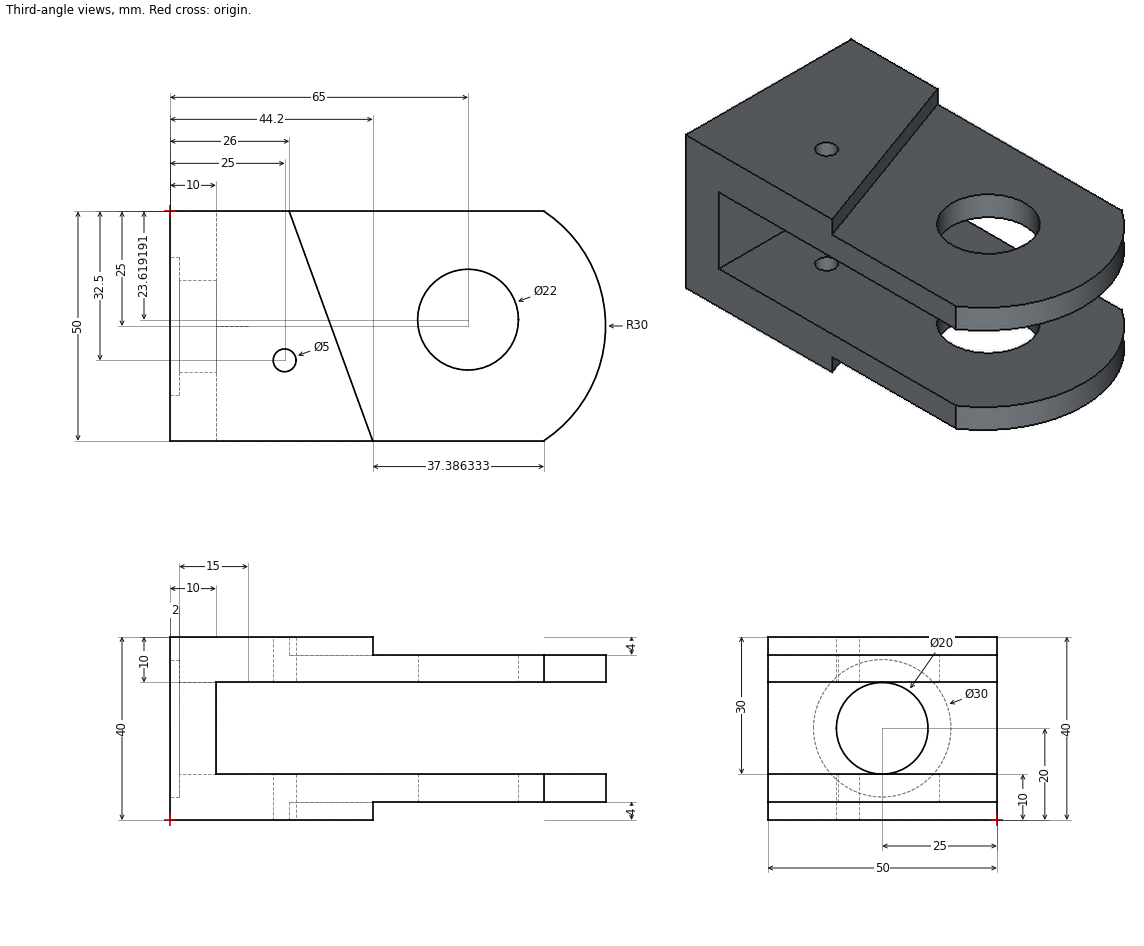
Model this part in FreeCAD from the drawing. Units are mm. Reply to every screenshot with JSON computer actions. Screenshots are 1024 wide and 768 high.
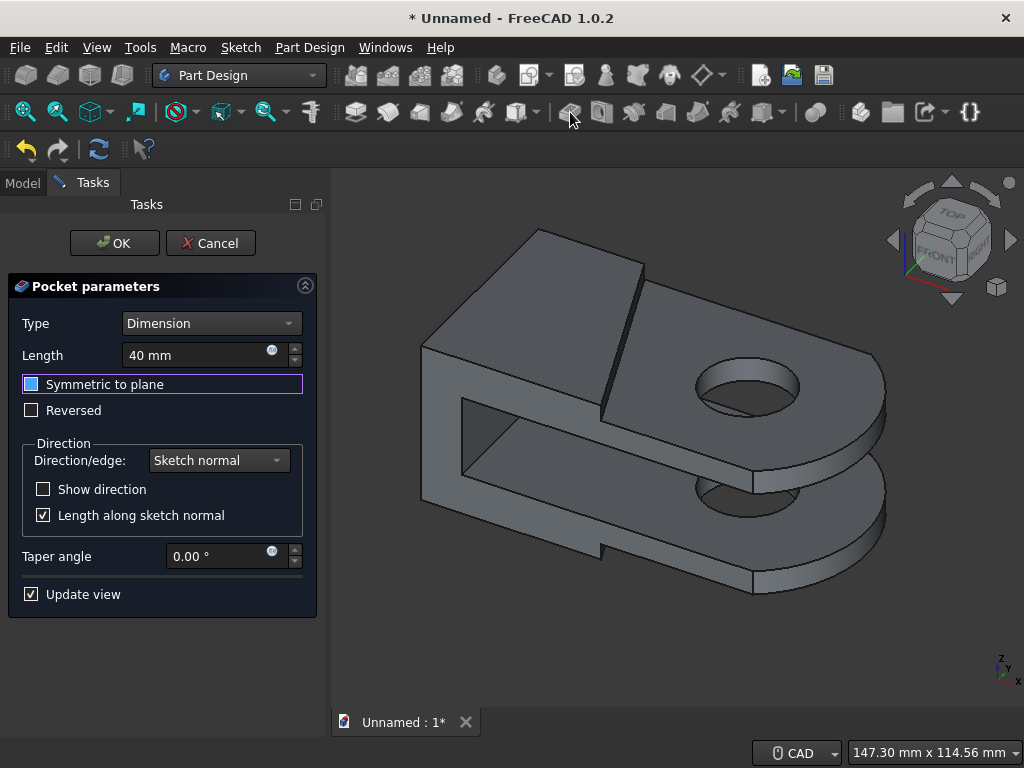
{"action": "left_click", "coordinate": [115, 243]}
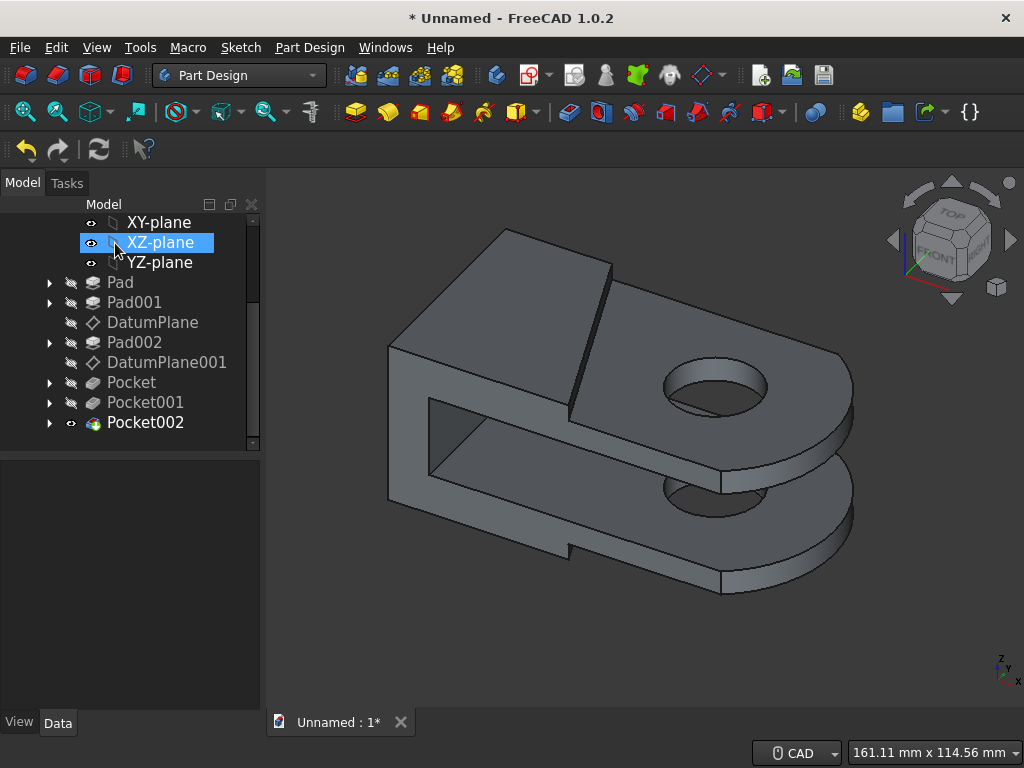
{"action": "left_click", "coordinate": [530, 76]}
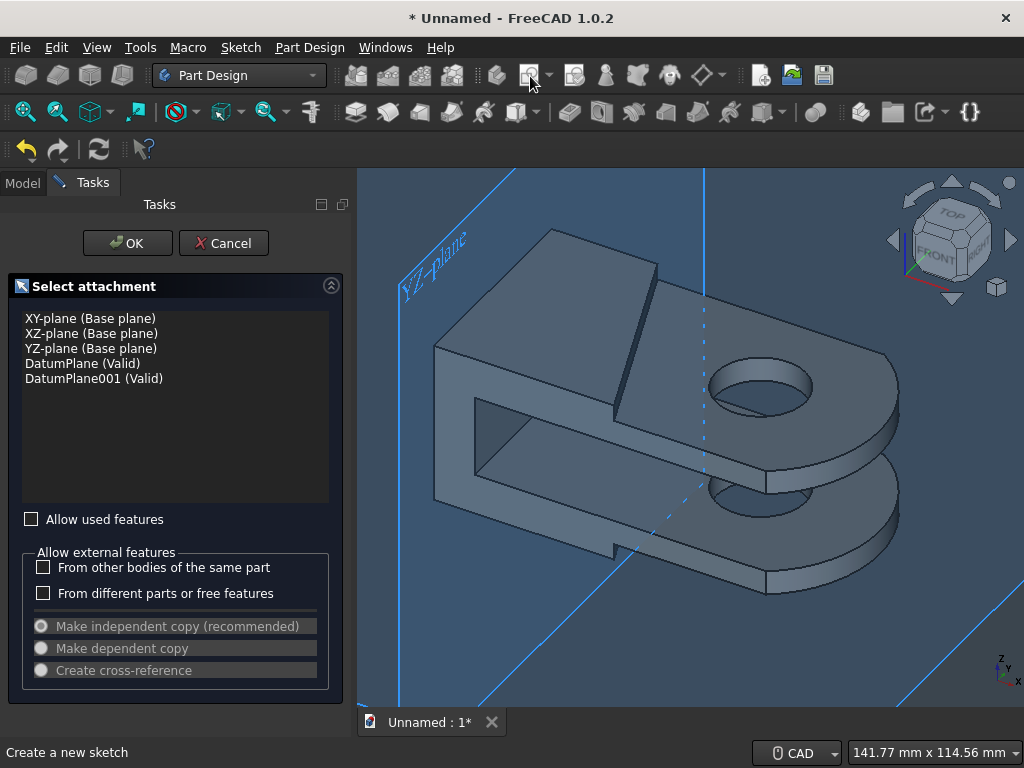
{"action": "left_click", "coordinate": [82, 348]}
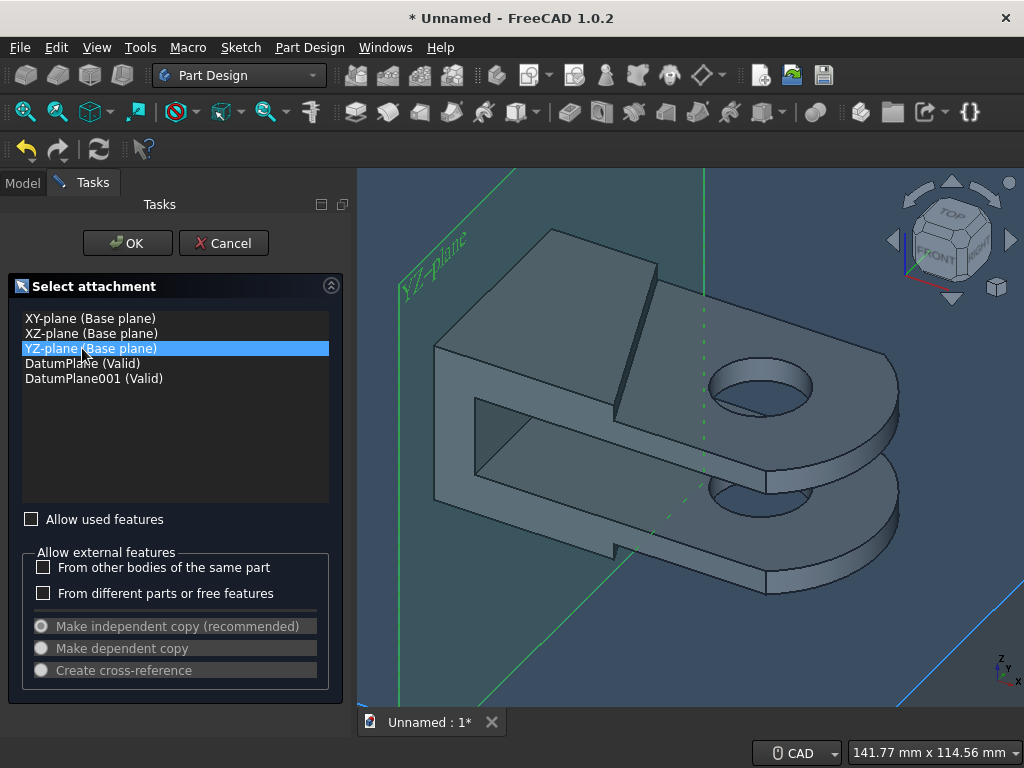
{"action": "left_click", "coordinate": [128, 243]}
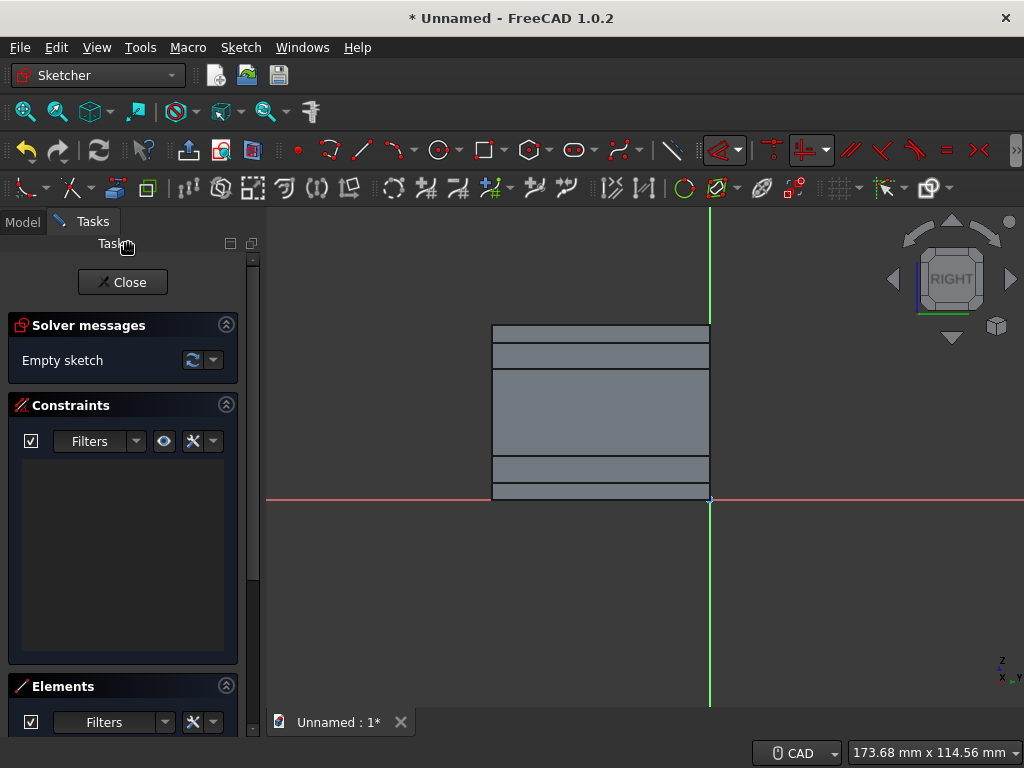
{"action": "key", "text": "q s"}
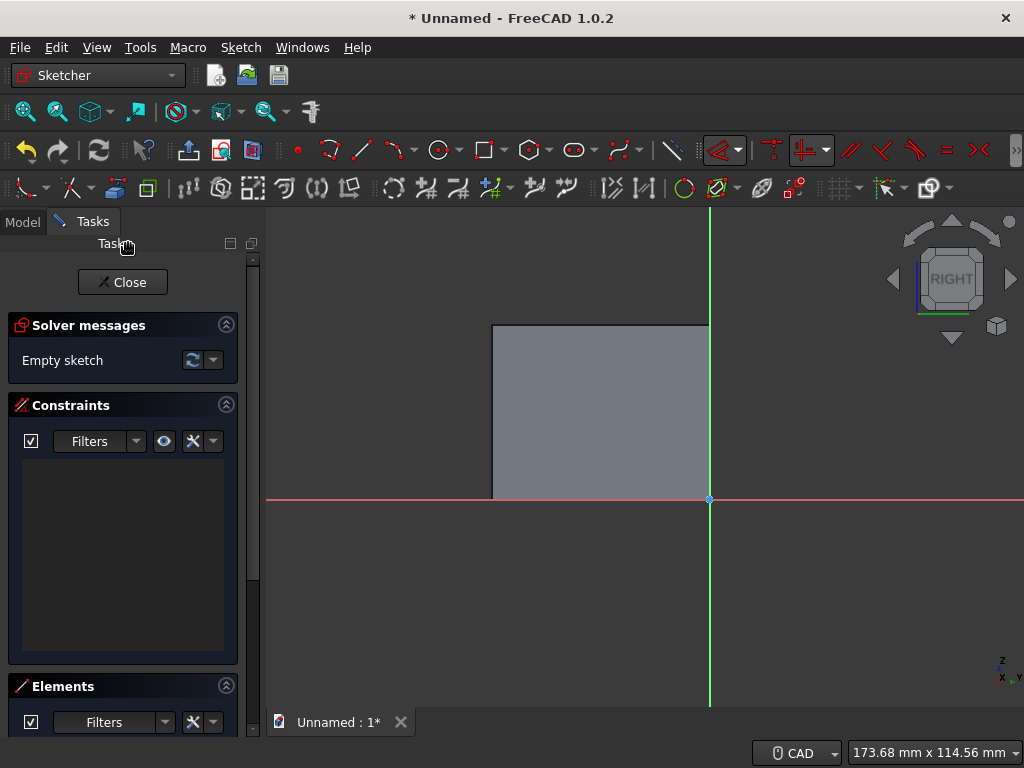
{"action": "scroll", "coordinate": [660, 396], "scroll_direction": "up", "scroll_amount": 4}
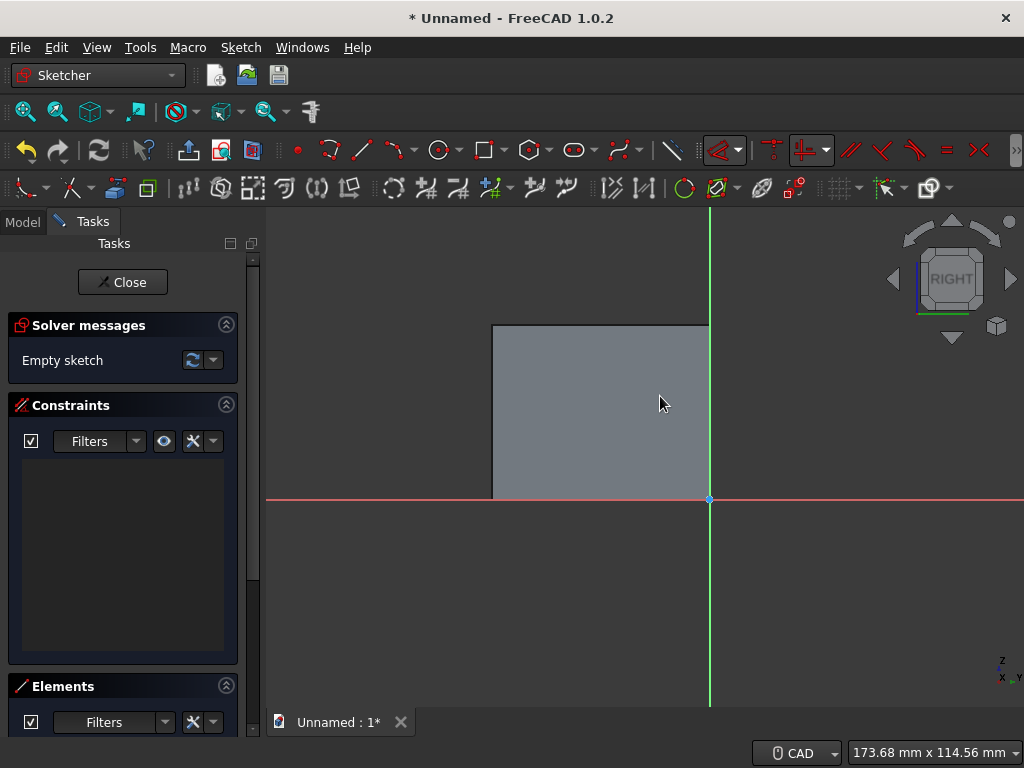
{"action": "left_click", "coordinate": [440, 150]}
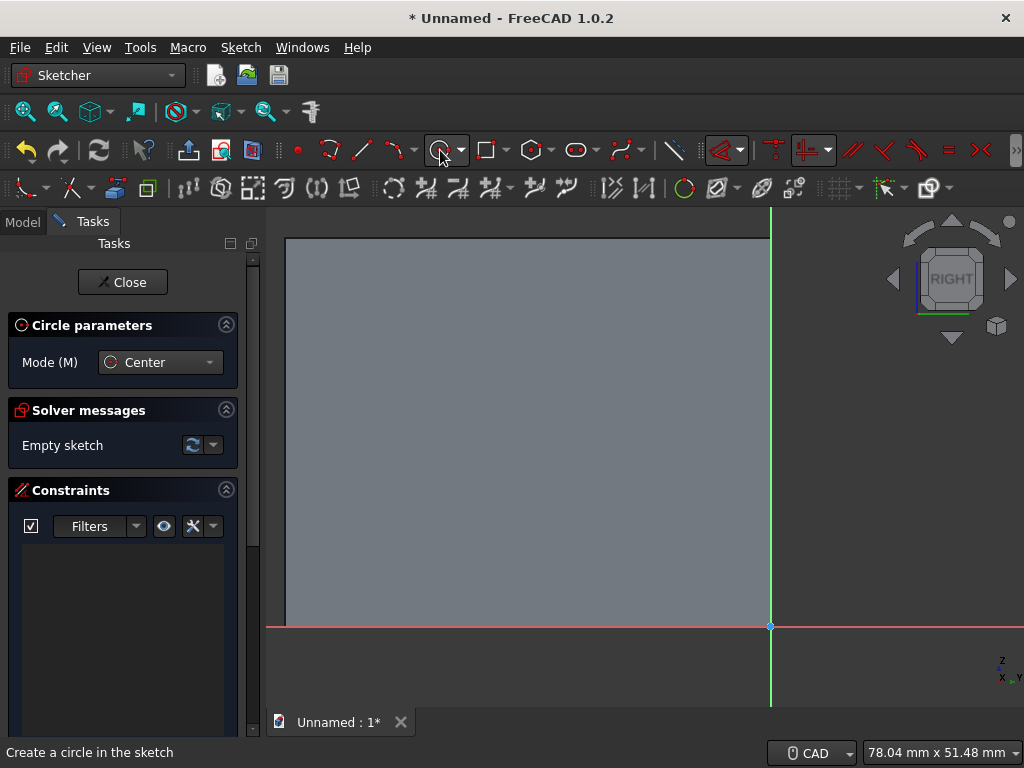
{"action": "left_click", "coordinate": [528, 433]}
{"action": "mouse_move", "coordinate": [631, 330]}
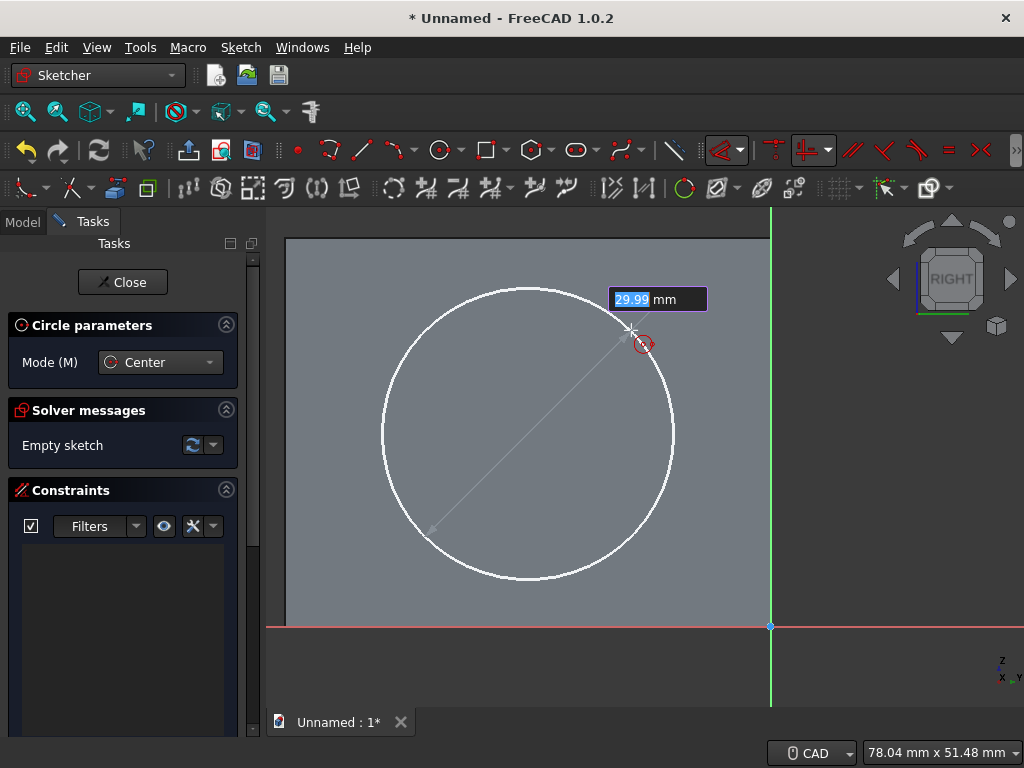
{"action": "type", "text": "30"}
{"action": "key", "text": "Return"}
{"action": "key", "text": "Escape"}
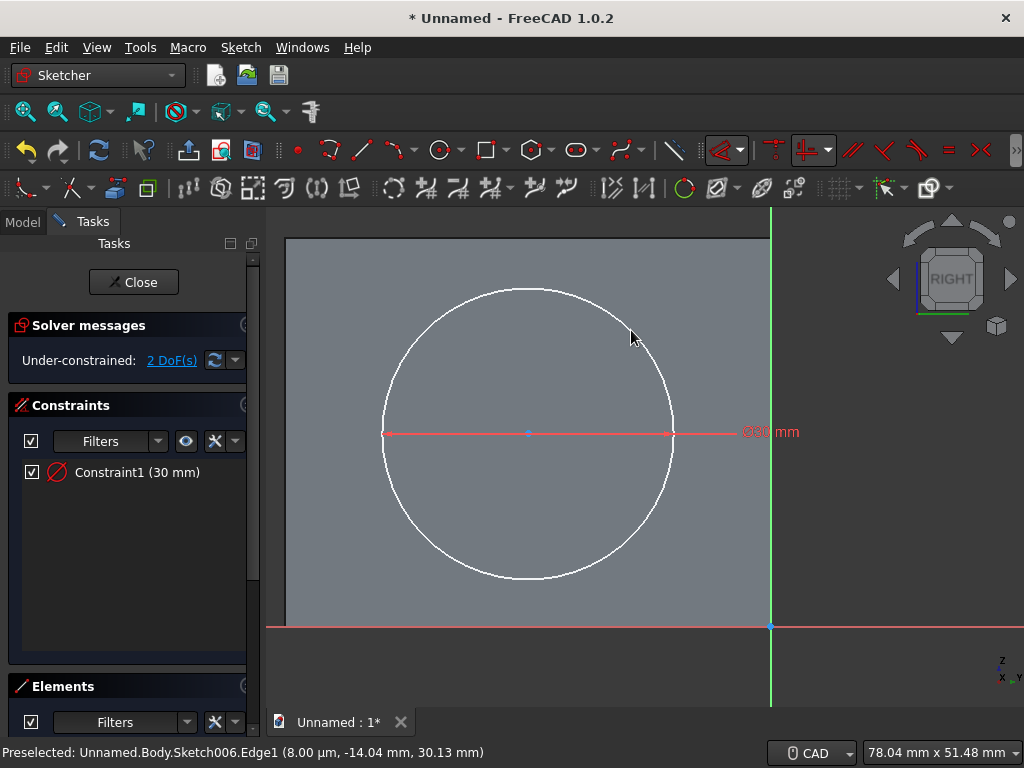
{"action": "left_click", "coordinate": [528, 434]}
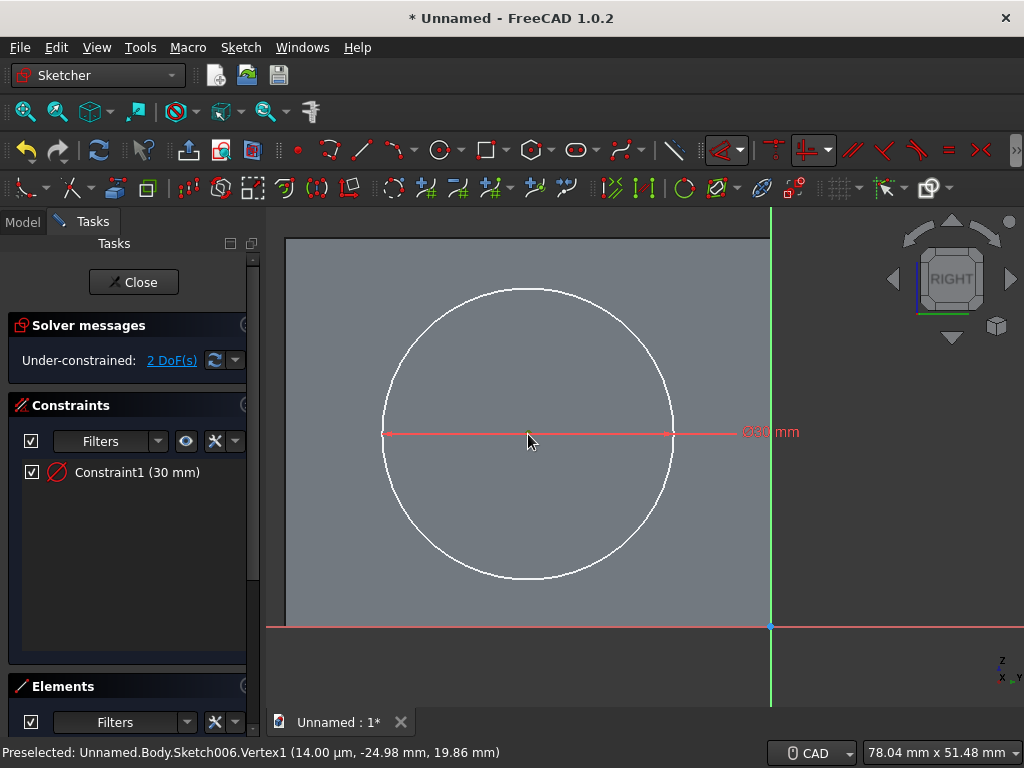
{"action": "left_click", "coordinate": [742, 150]}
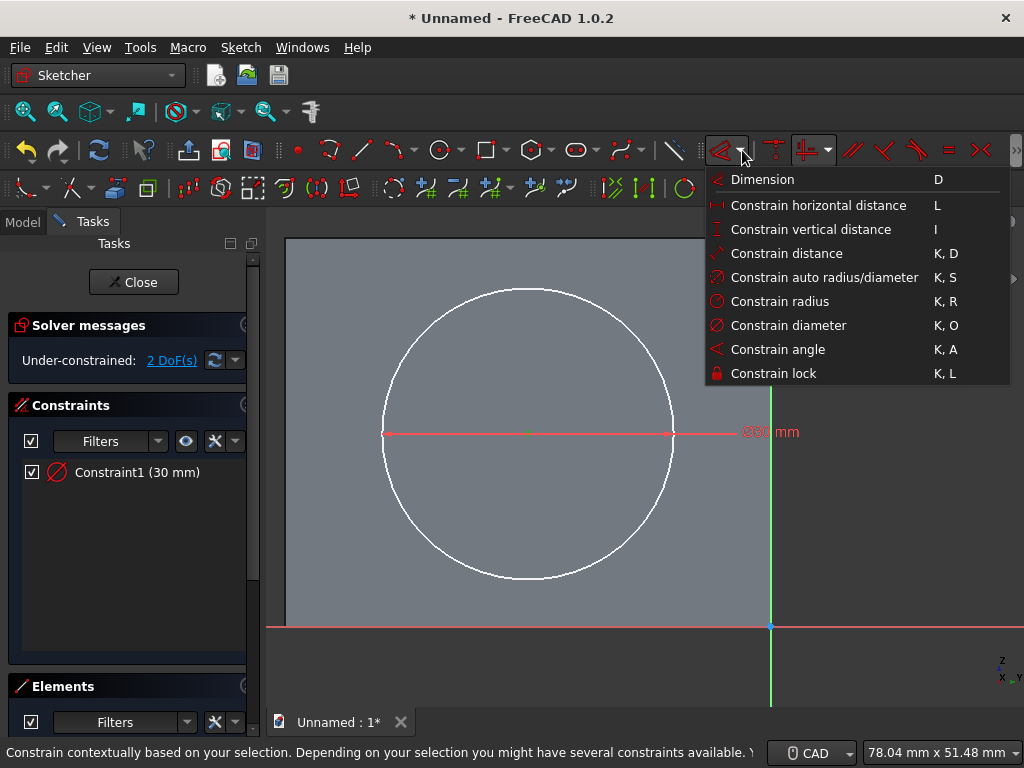
{"action": "left_click", "coordinate": [858, 205]}